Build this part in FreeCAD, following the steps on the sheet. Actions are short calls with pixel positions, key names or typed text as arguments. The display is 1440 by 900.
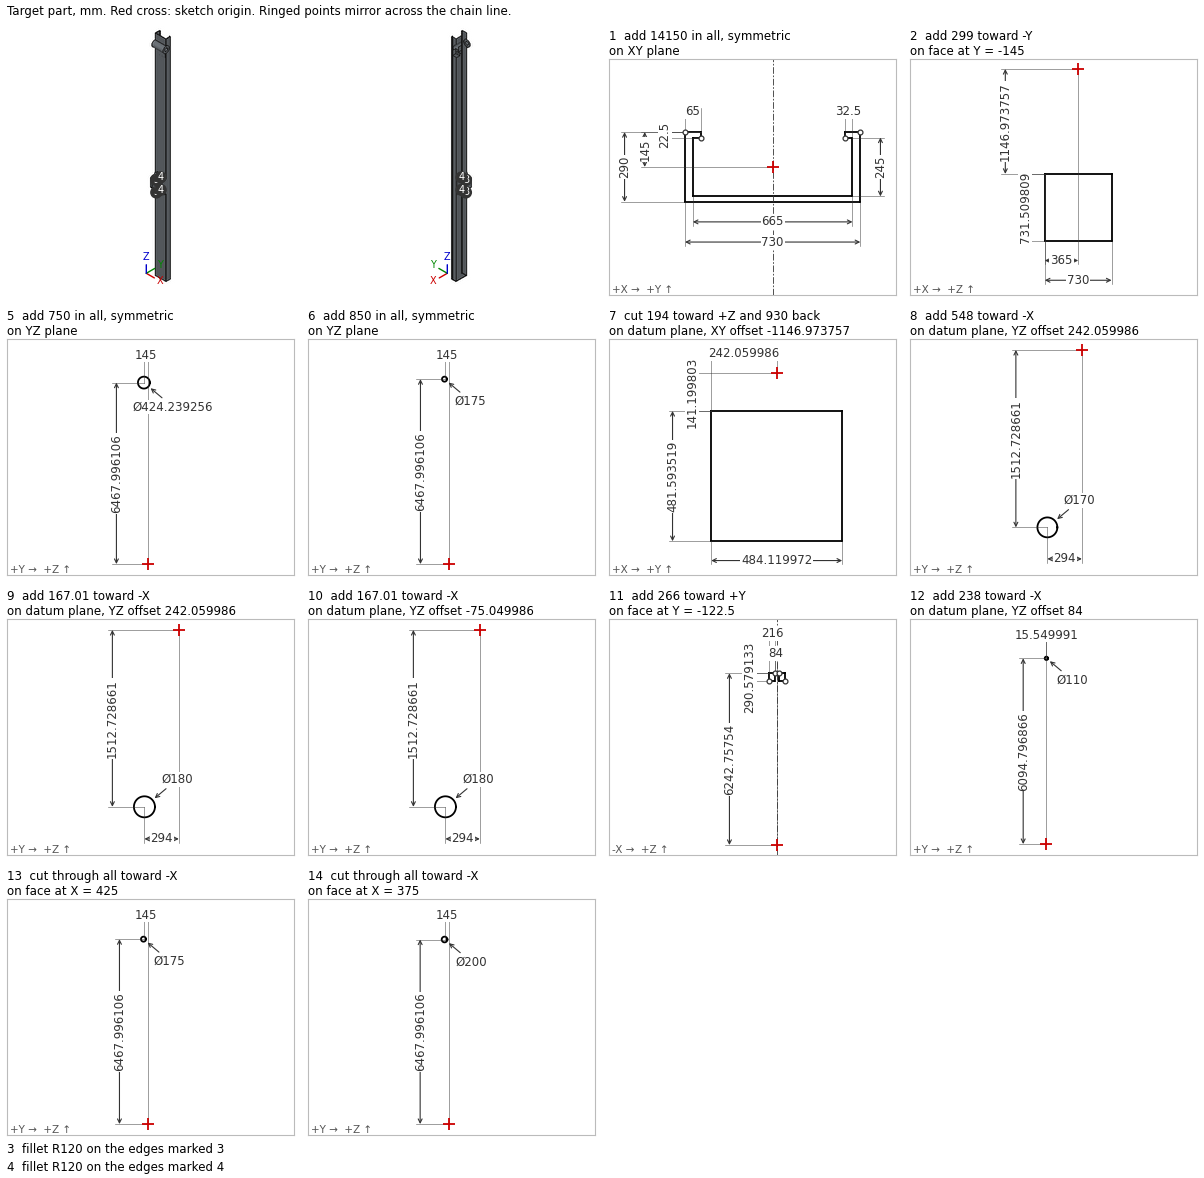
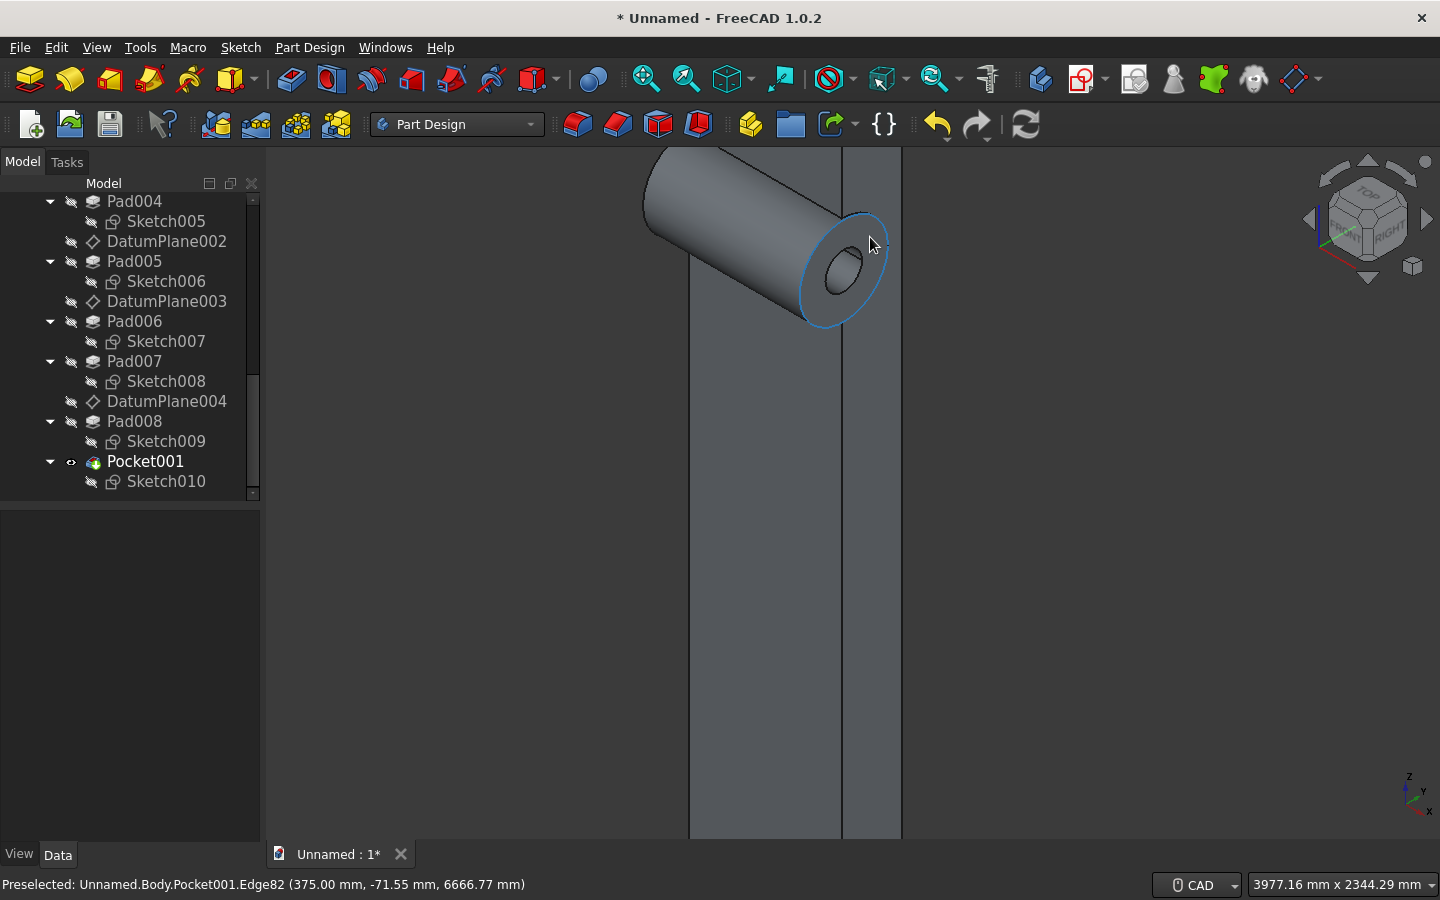
click(869, 241)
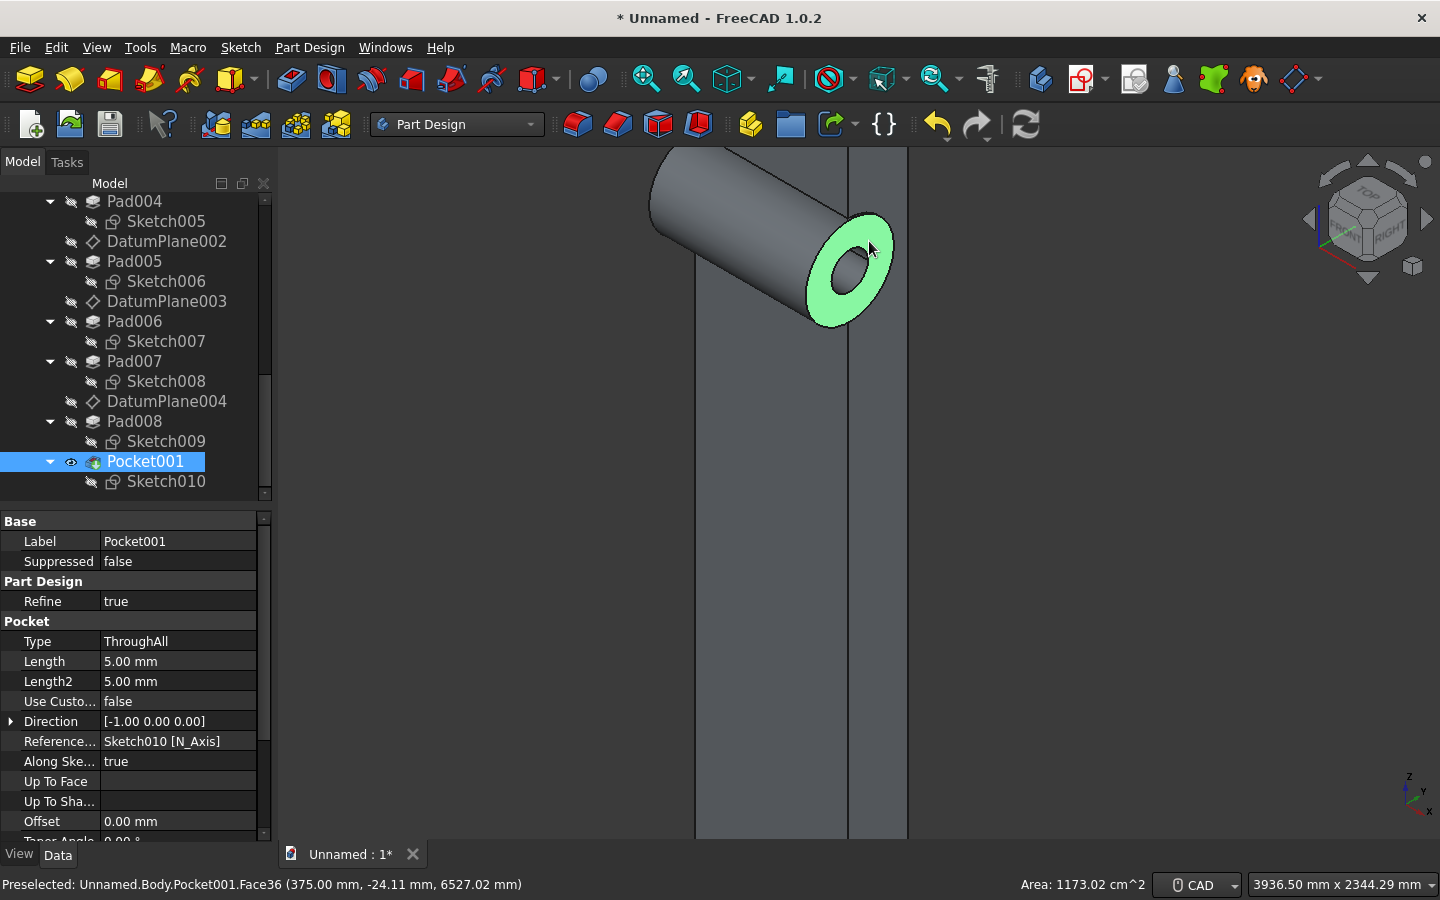
click(1082, 80)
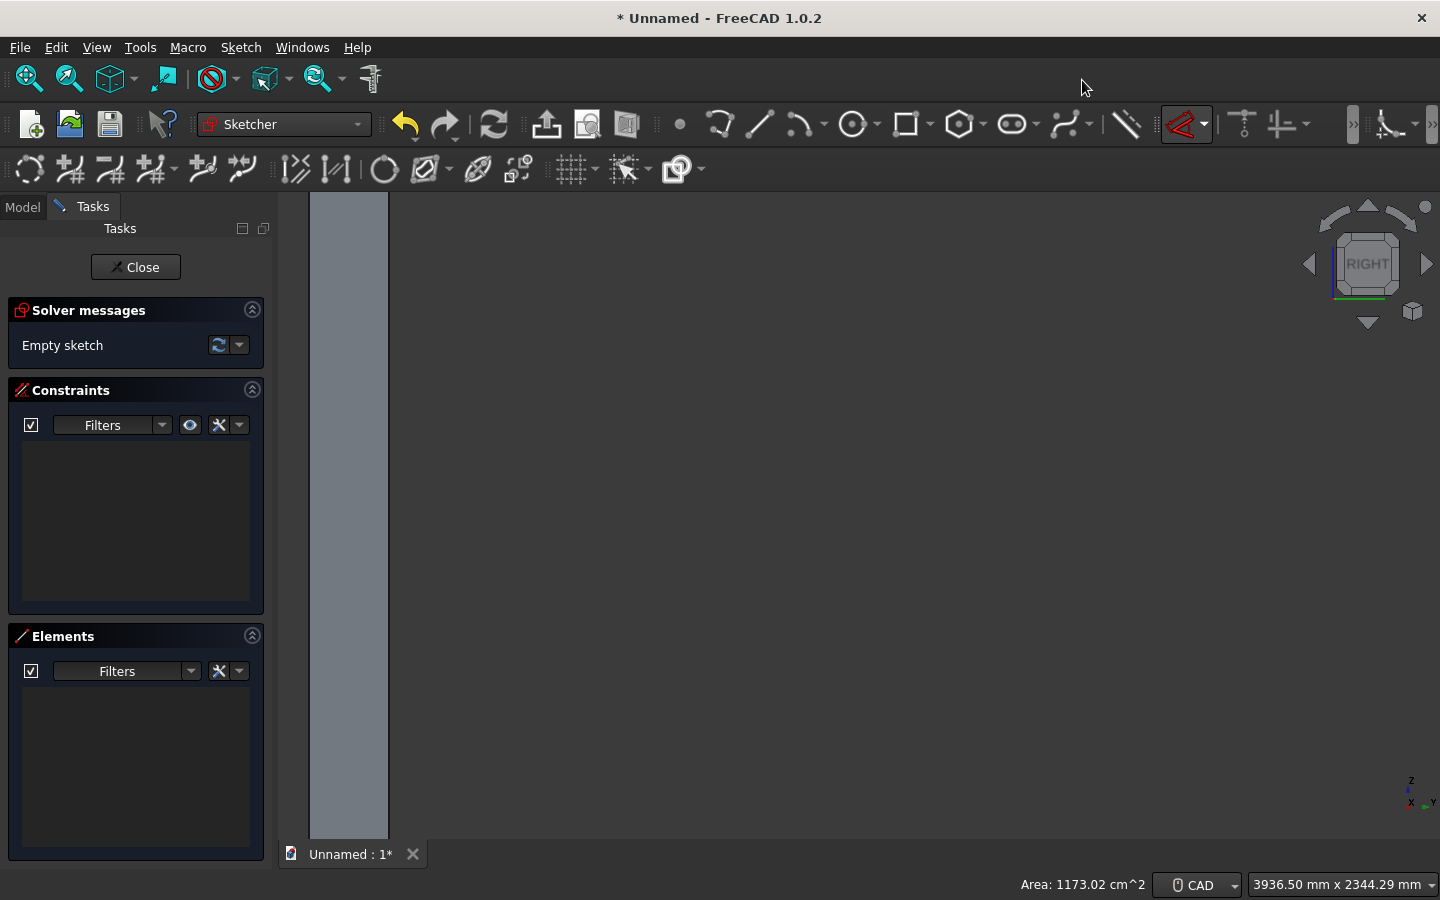
scroll(784, 516, down, 5)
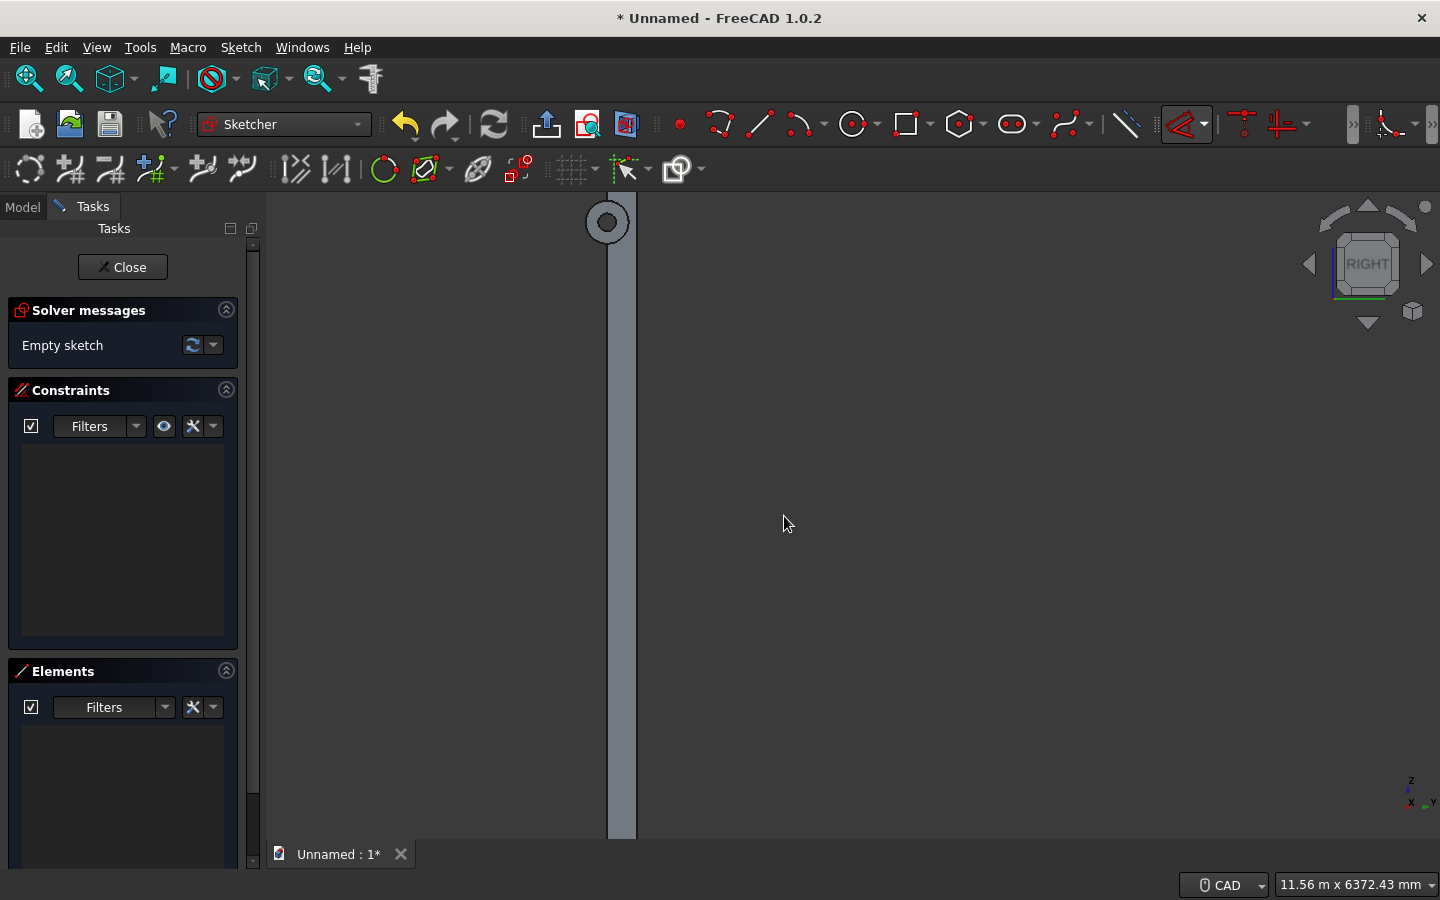
scroll(784, 516, down, 5)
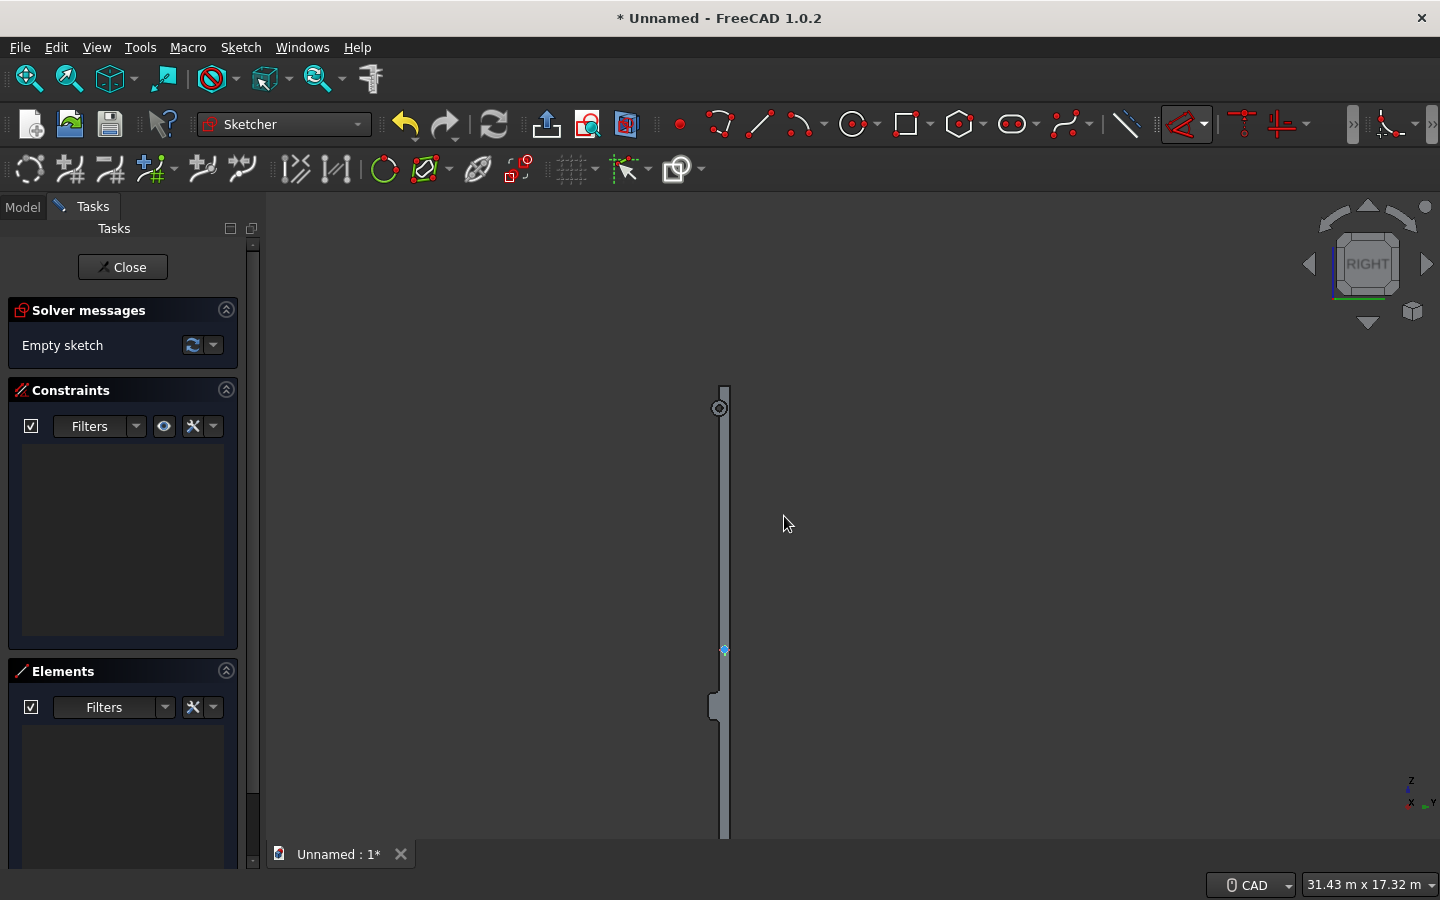
scroll(716, 403, up, 15)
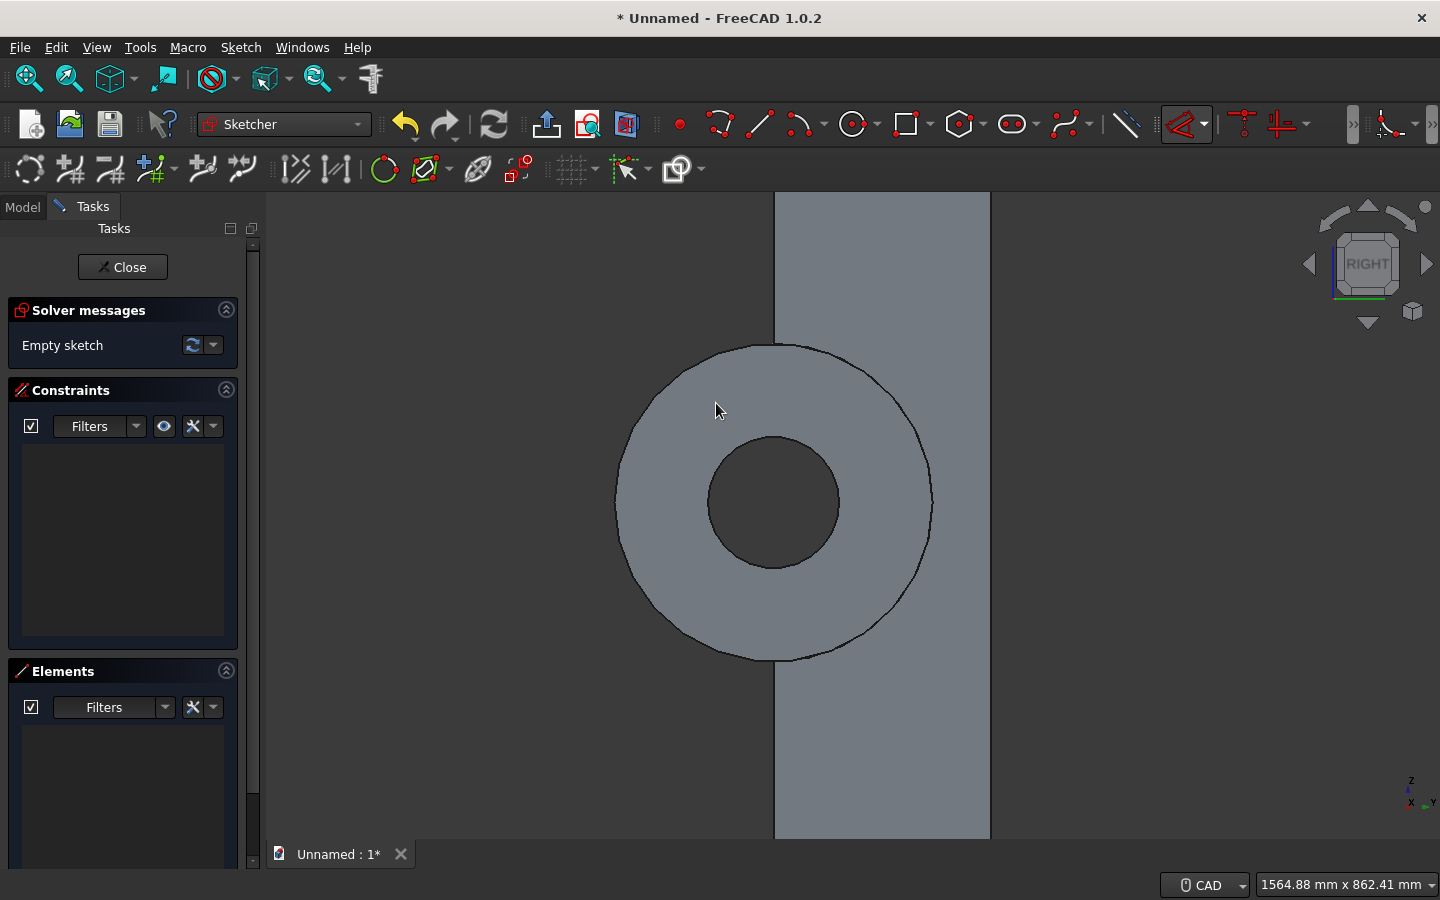
scroll(767, 495, up, 5)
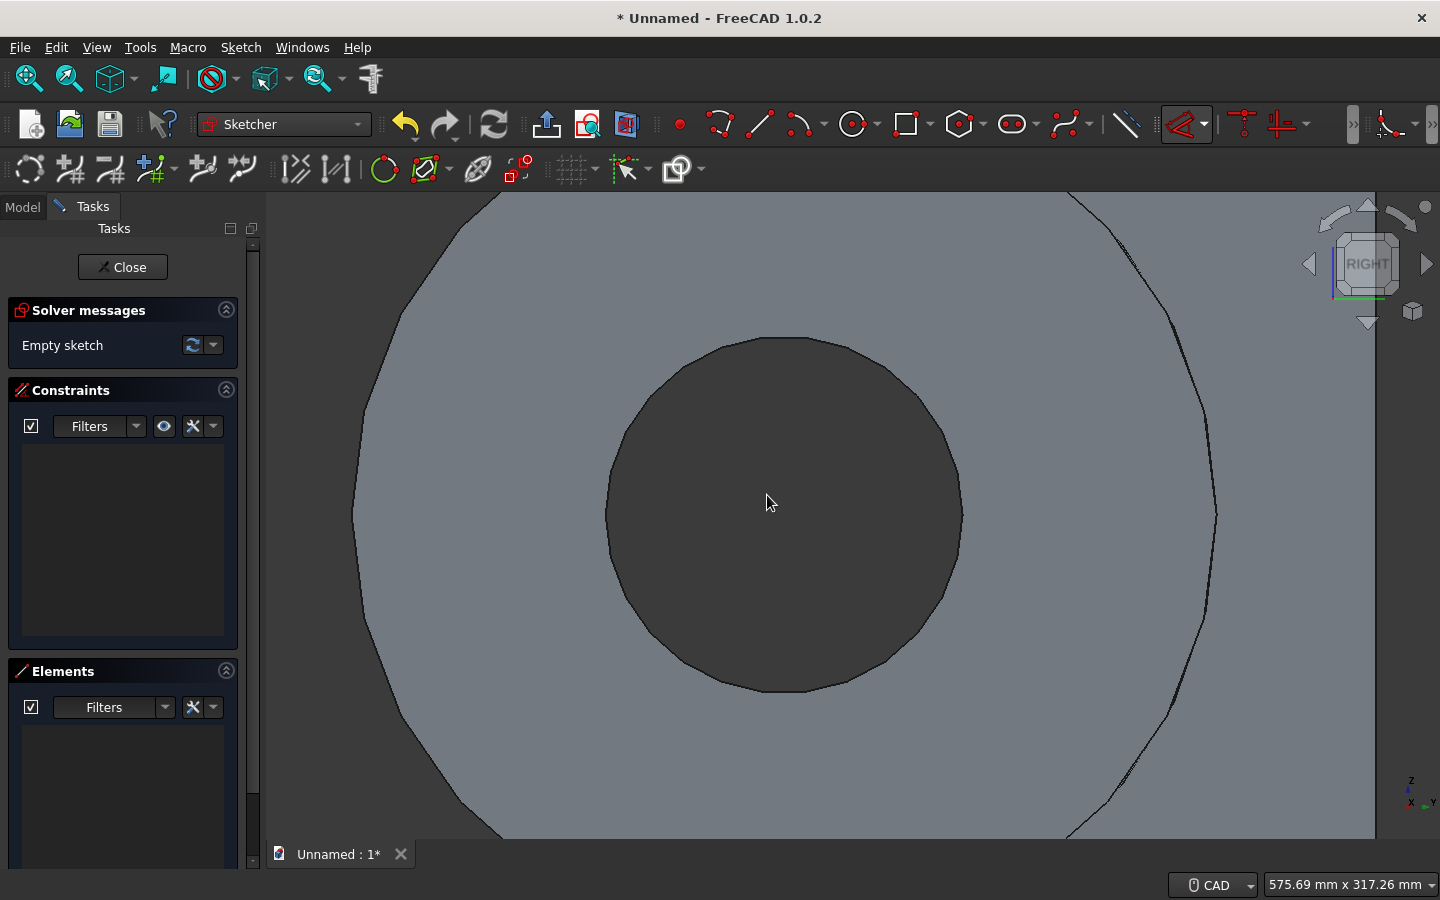
key(g)
key(c)